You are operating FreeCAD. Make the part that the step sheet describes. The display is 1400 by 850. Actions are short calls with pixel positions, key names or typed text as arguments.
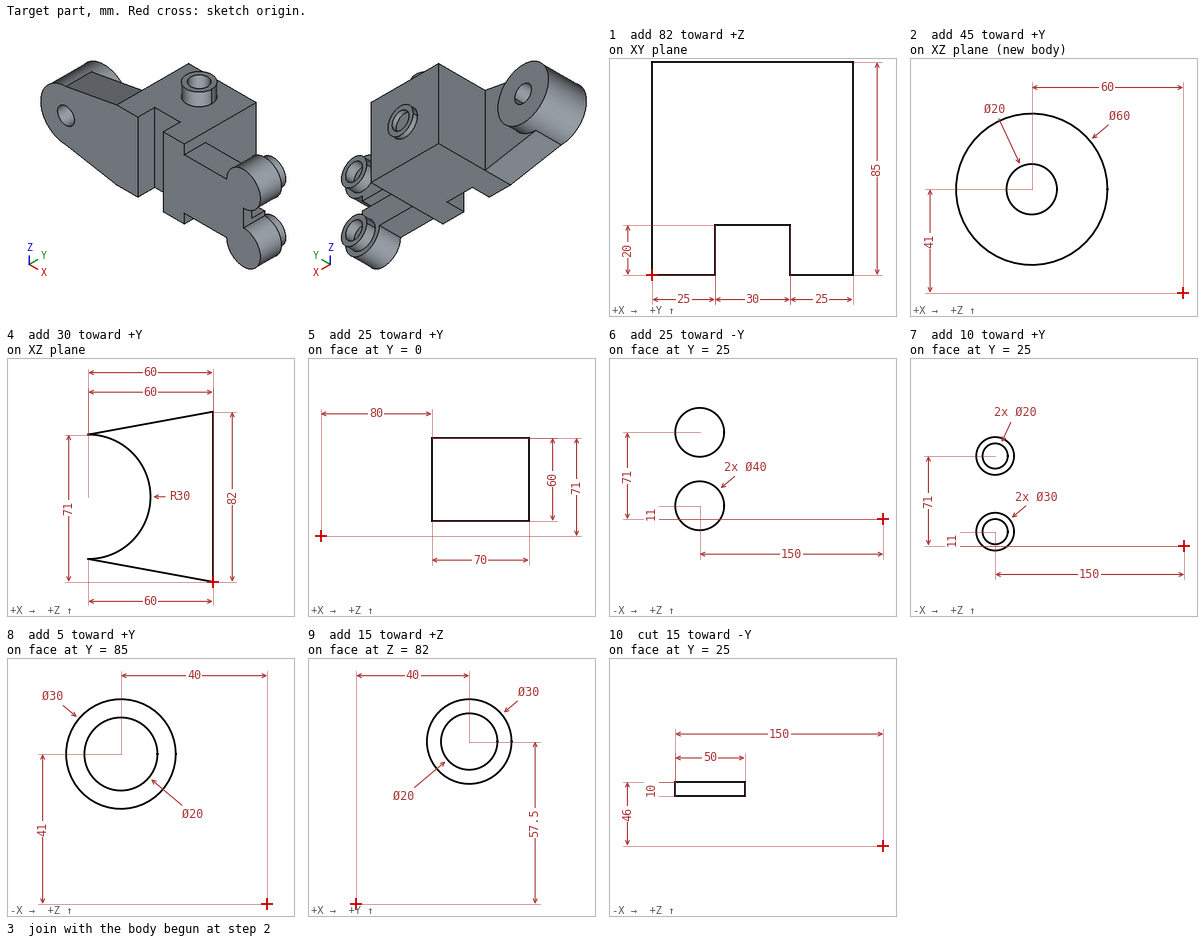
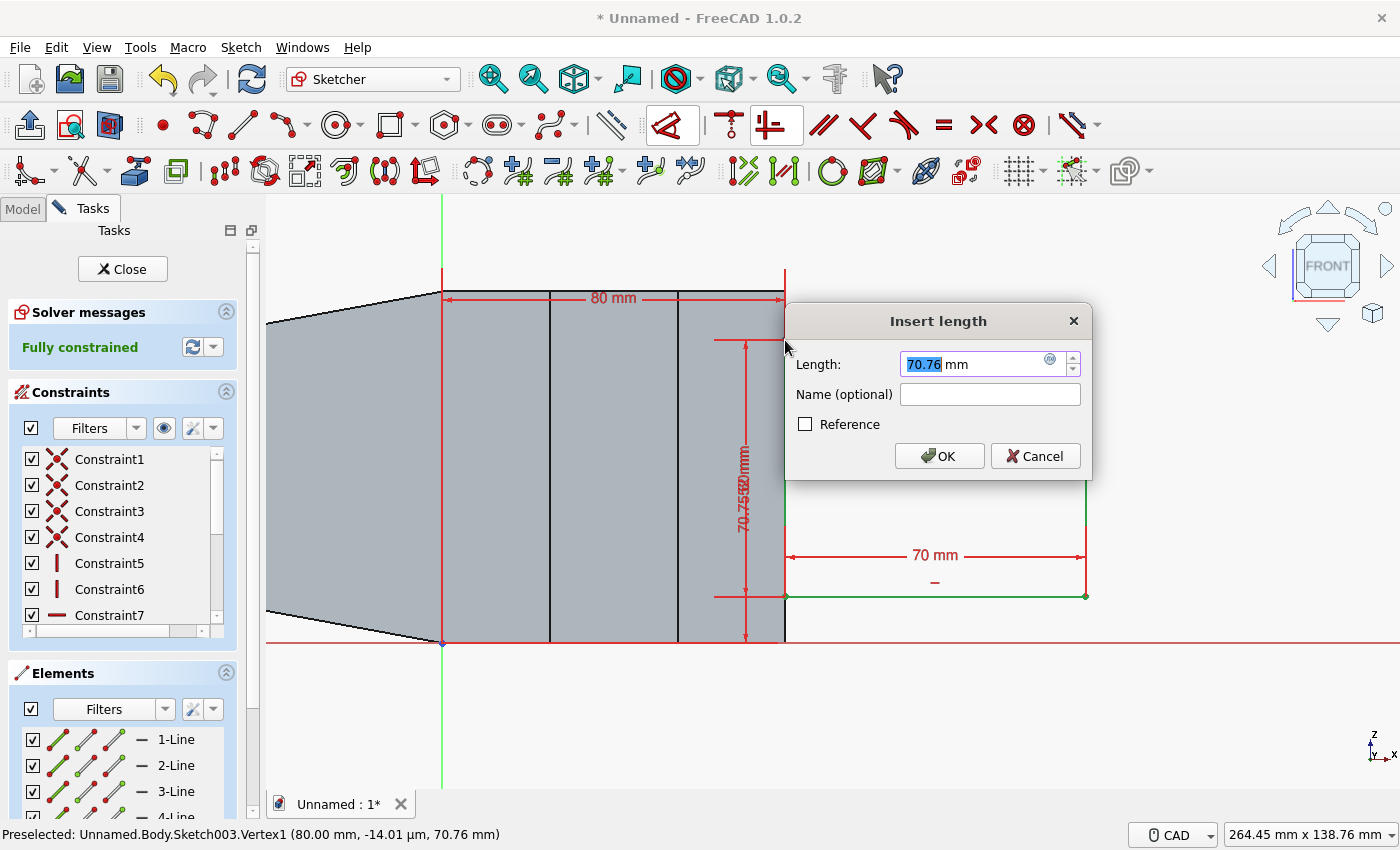
text(71)
key(Return)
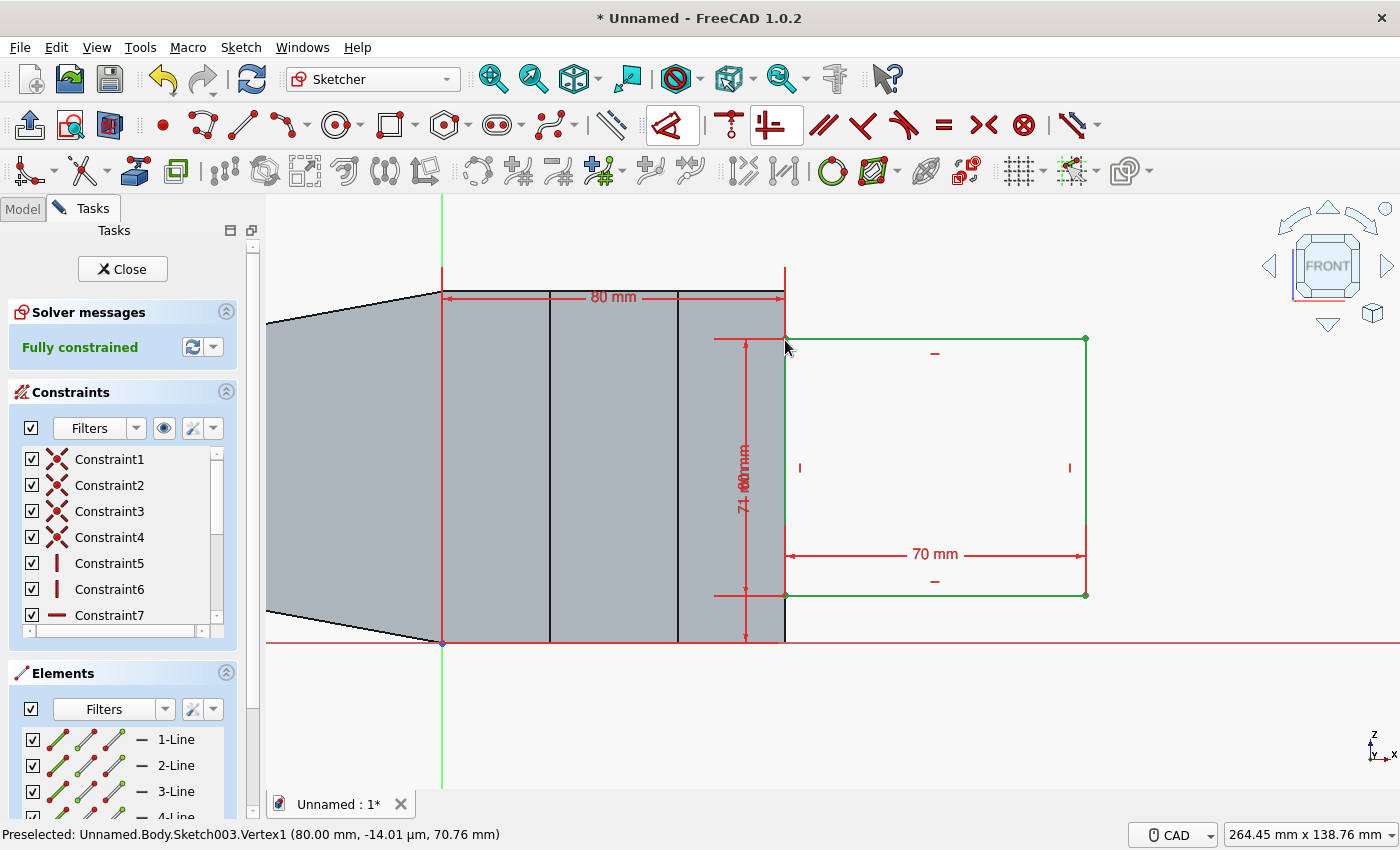
click(123, 269)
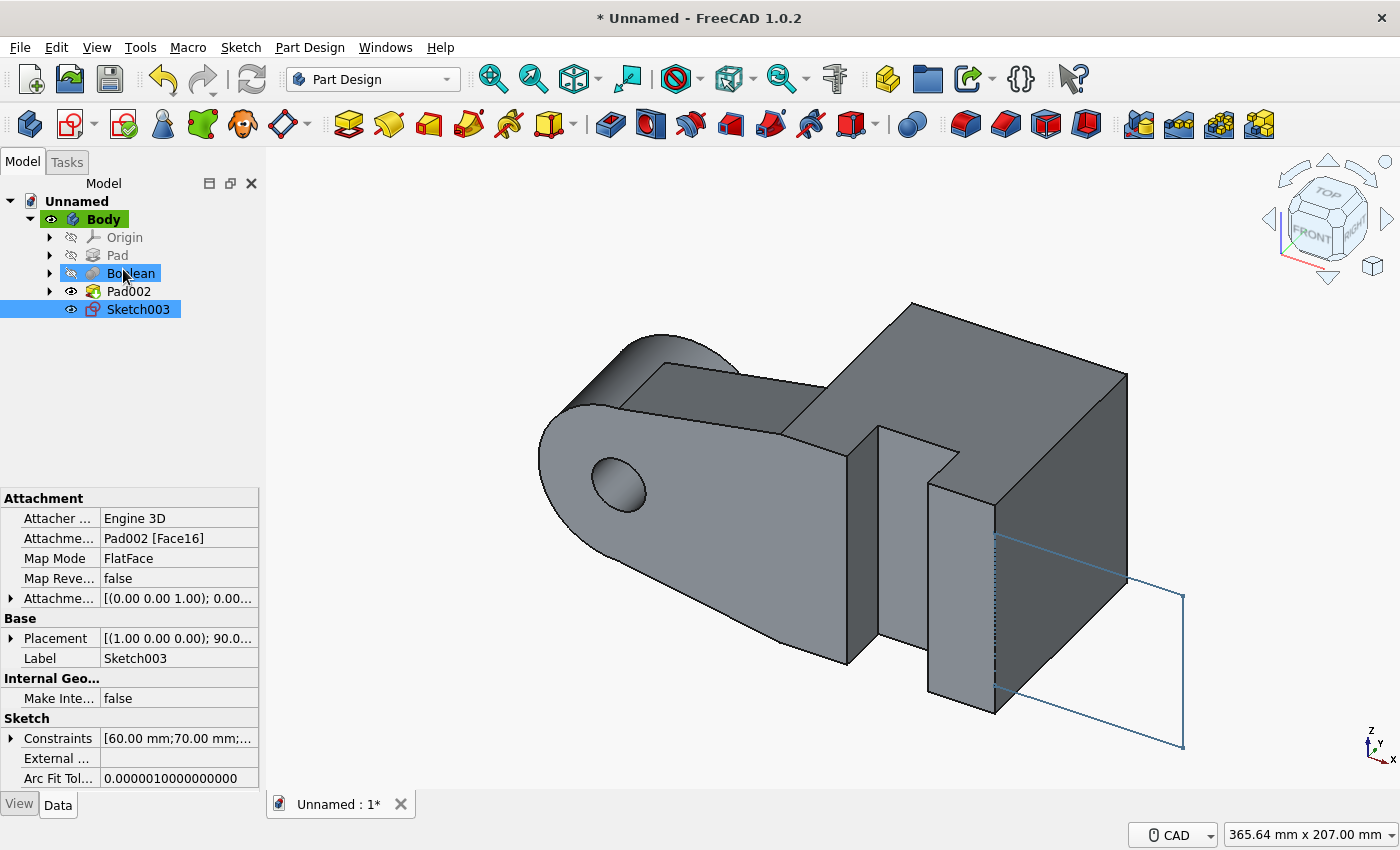
click(350, 124)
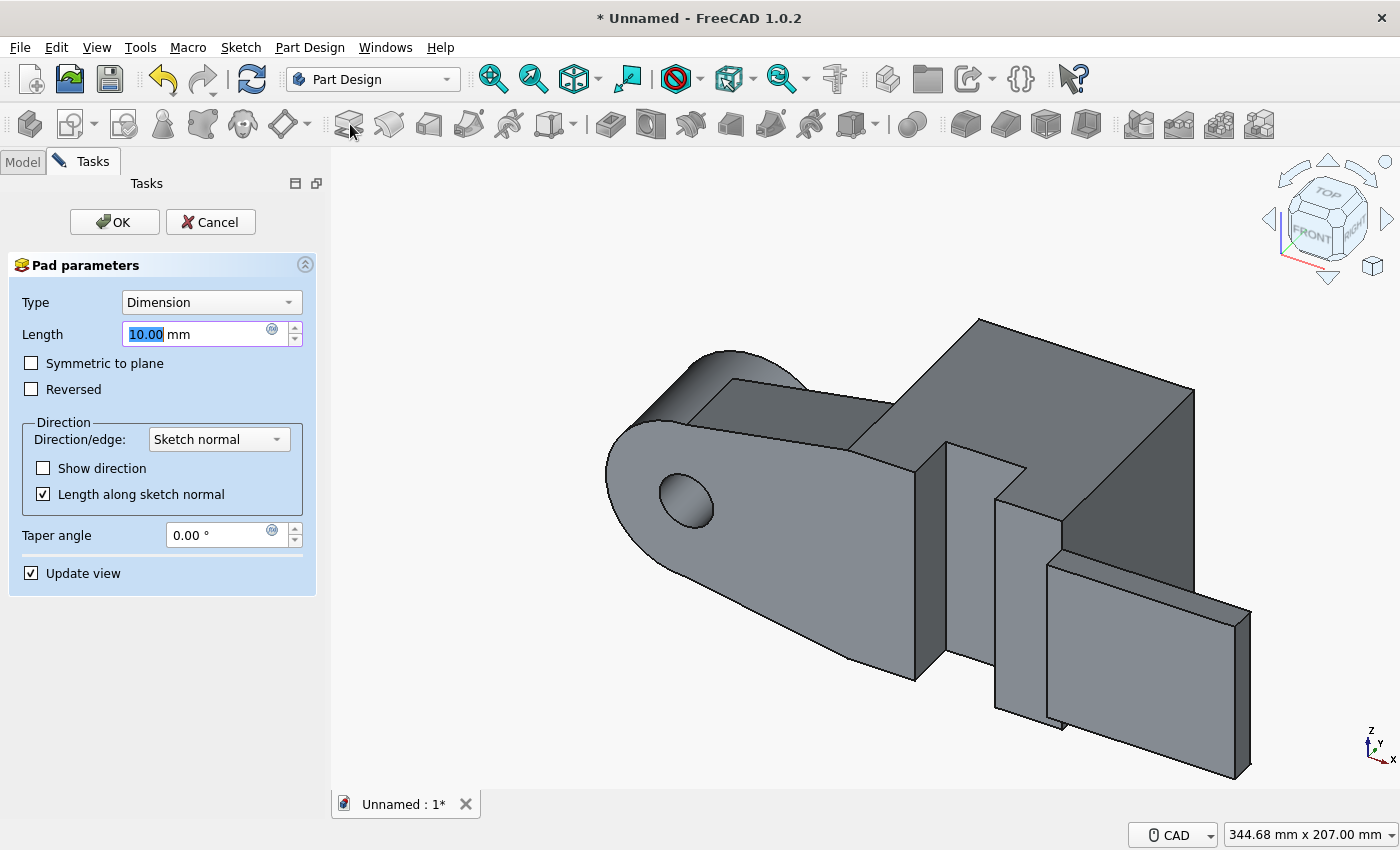
text(25)
key(Tab)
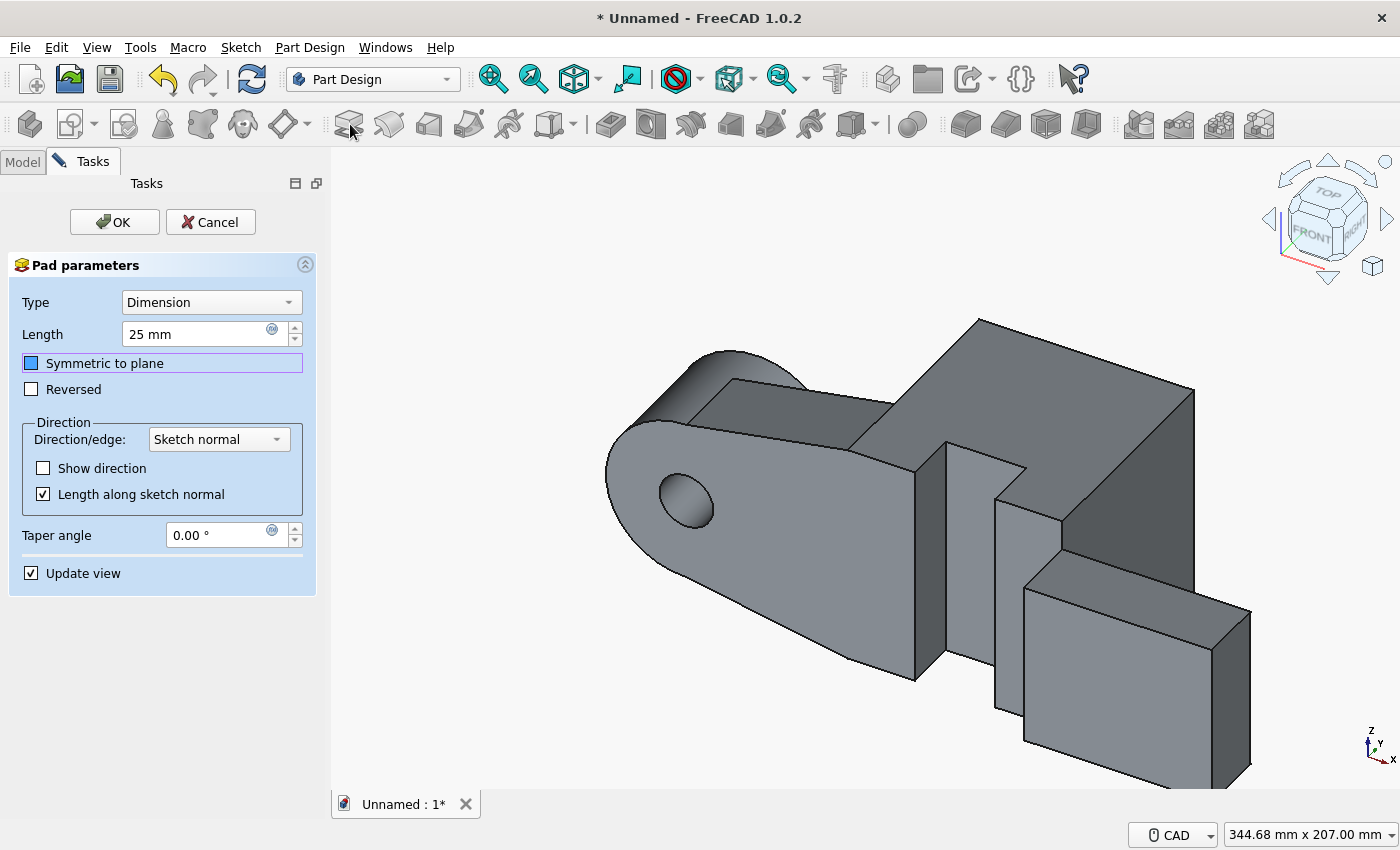
click(30, 389)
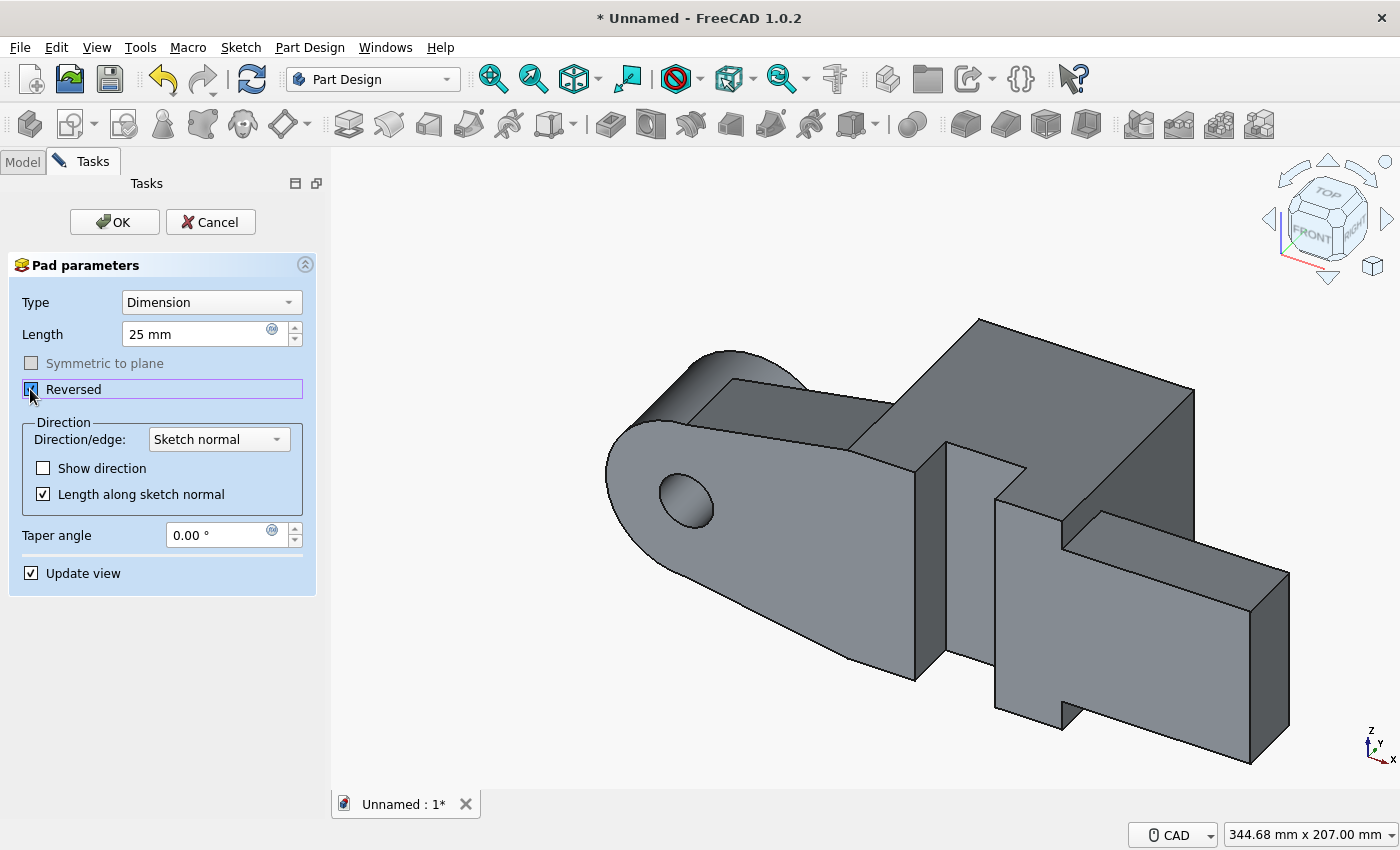
click(115, 222)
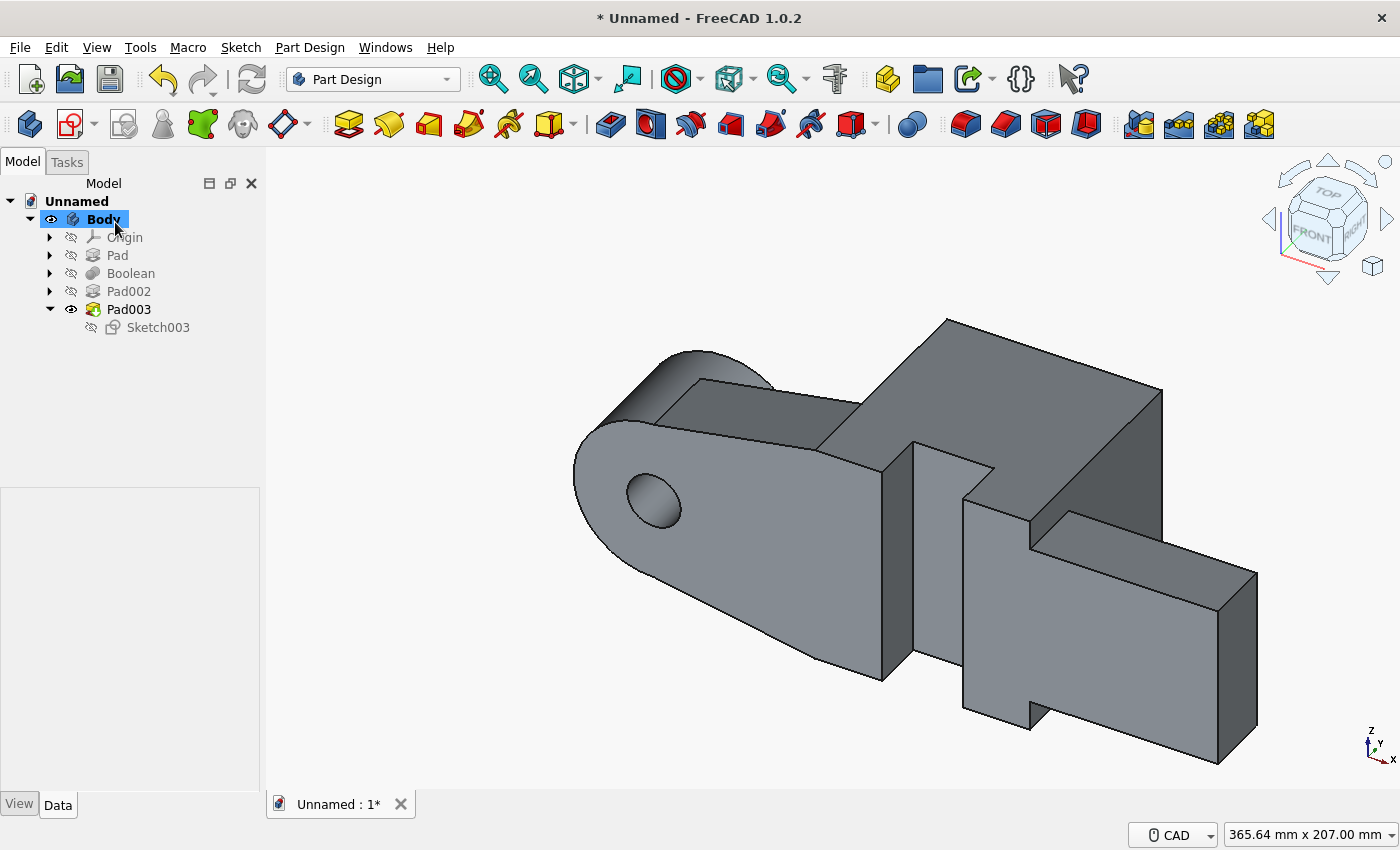
click(494, 80)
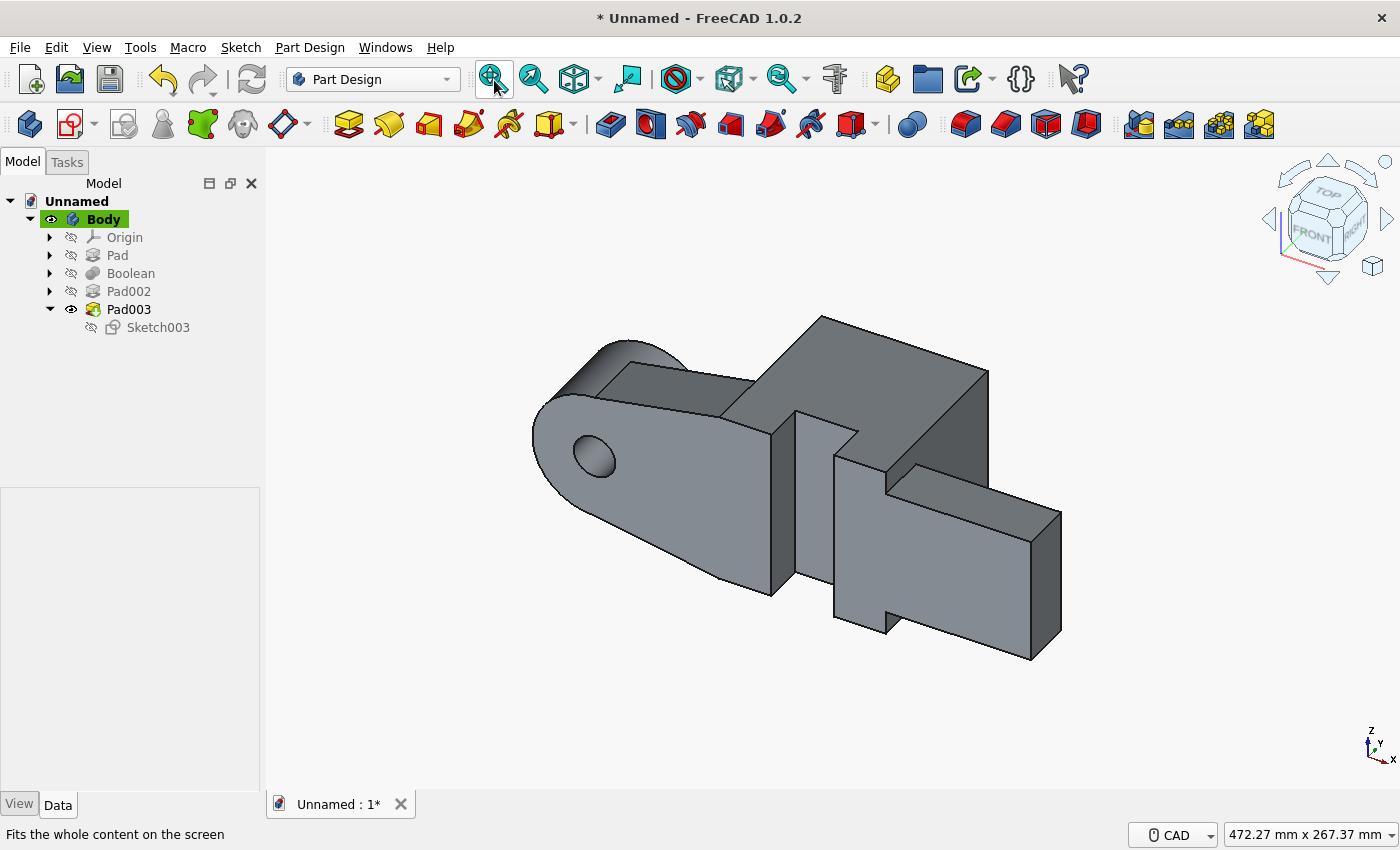
key(4)